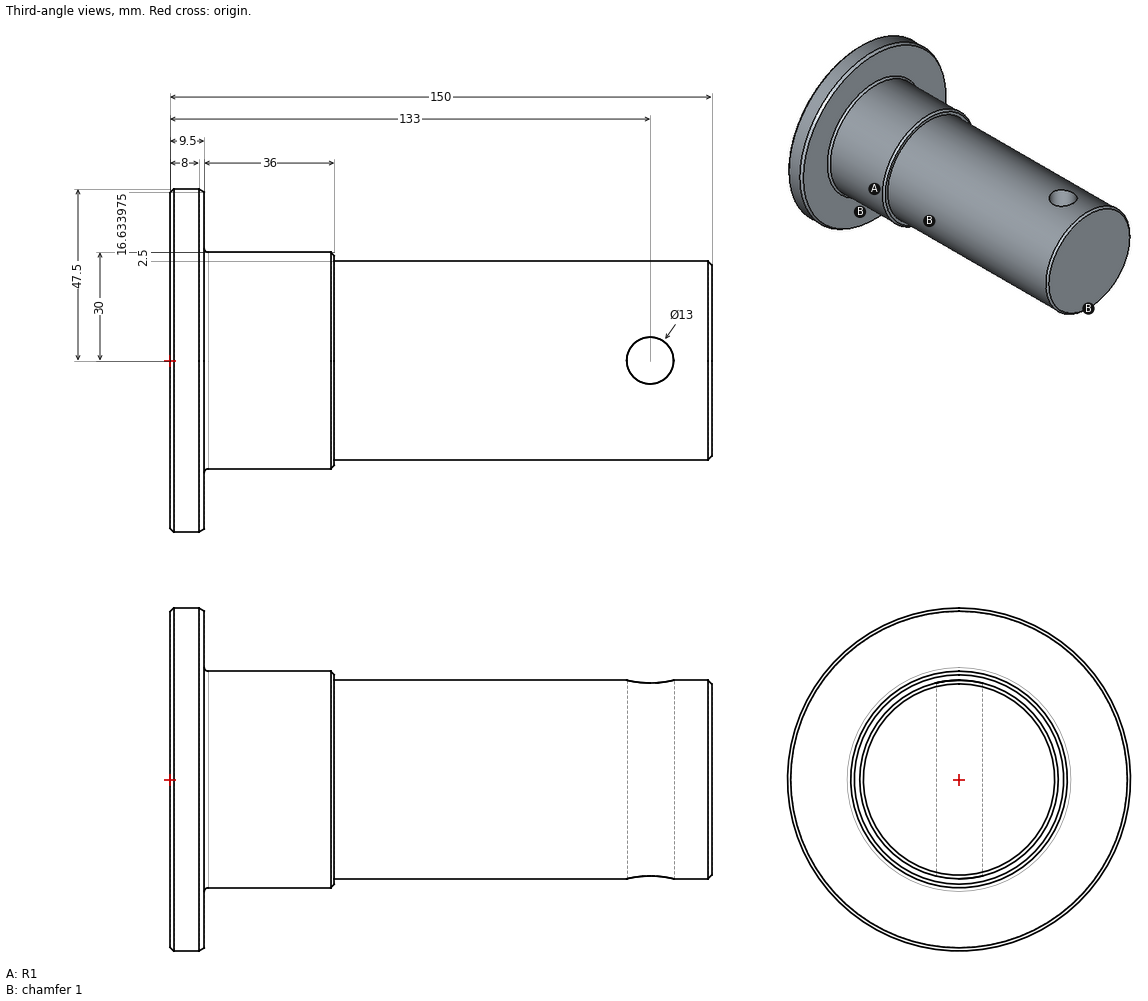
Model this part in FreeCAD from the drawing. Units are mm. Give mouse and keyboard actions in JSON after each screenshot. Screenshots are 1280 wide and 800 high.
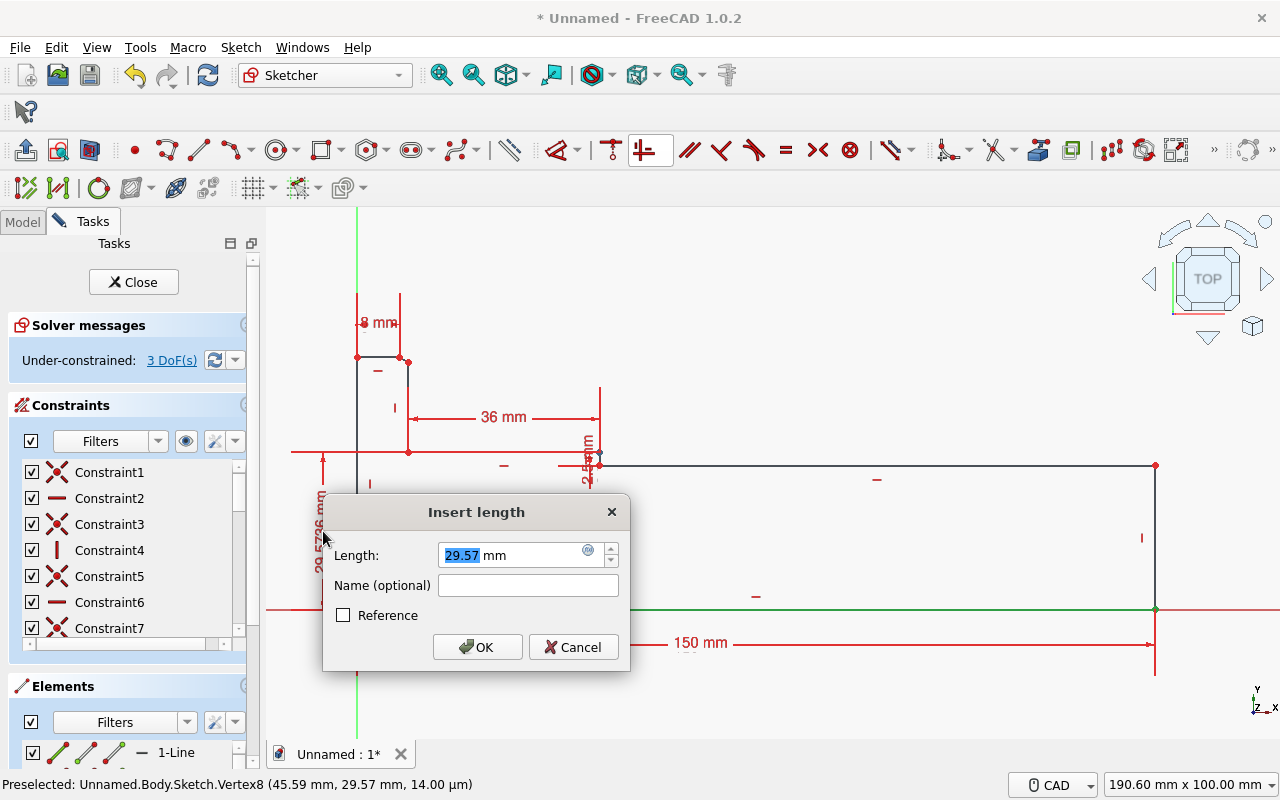
{"action": "type", "text": "30"}
{"action": "key", "text": "Return"}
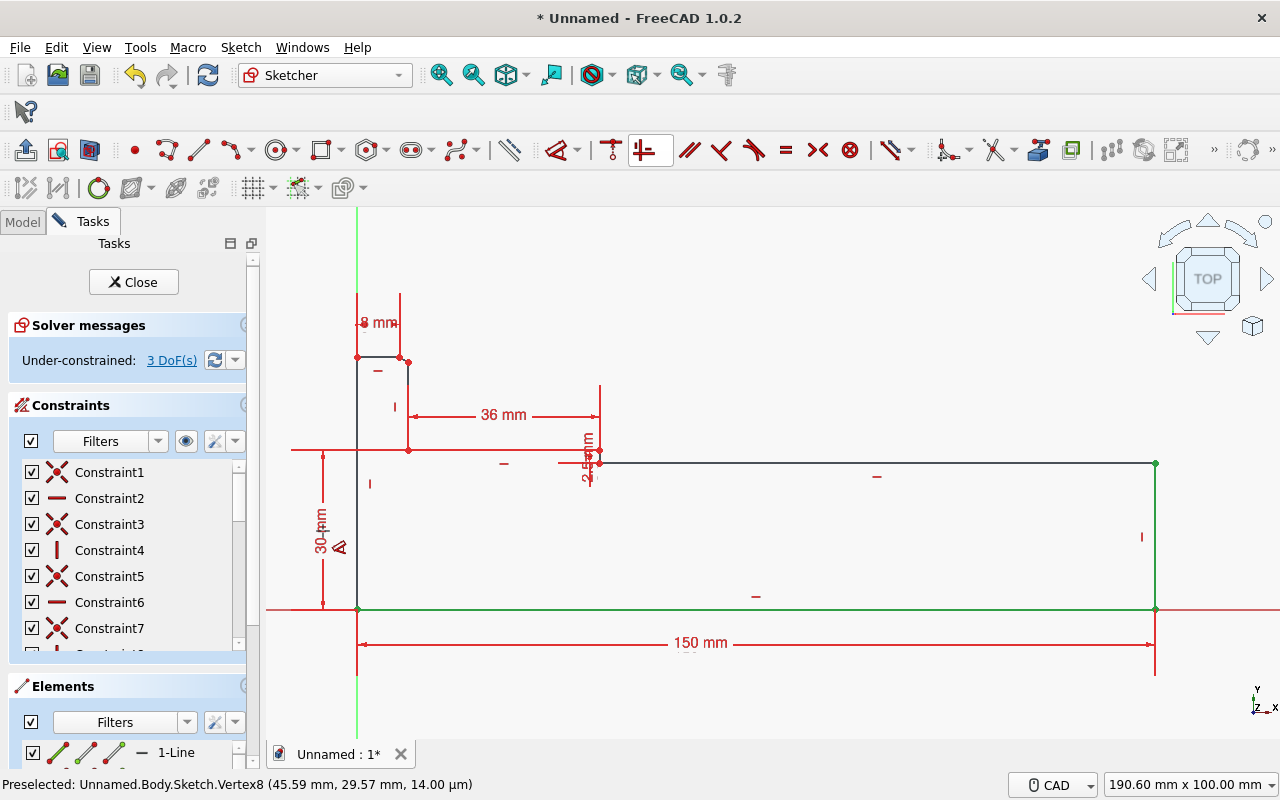
{"action": "left_click", "coordinate": [357, 433]}
{"action": "left_click", "coordinate": [323, 484]}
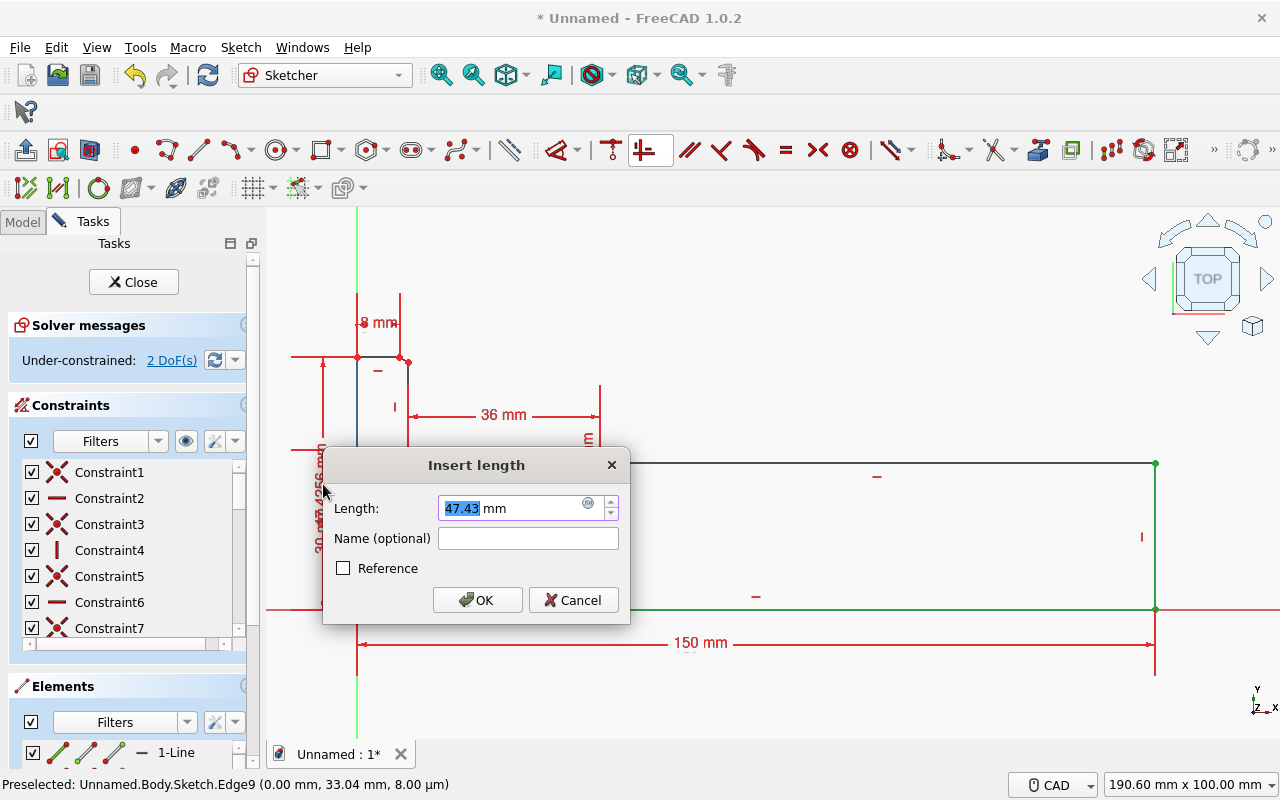
{"action": "type", "text": "47.5"}
{"action": "key", "text": "Return"}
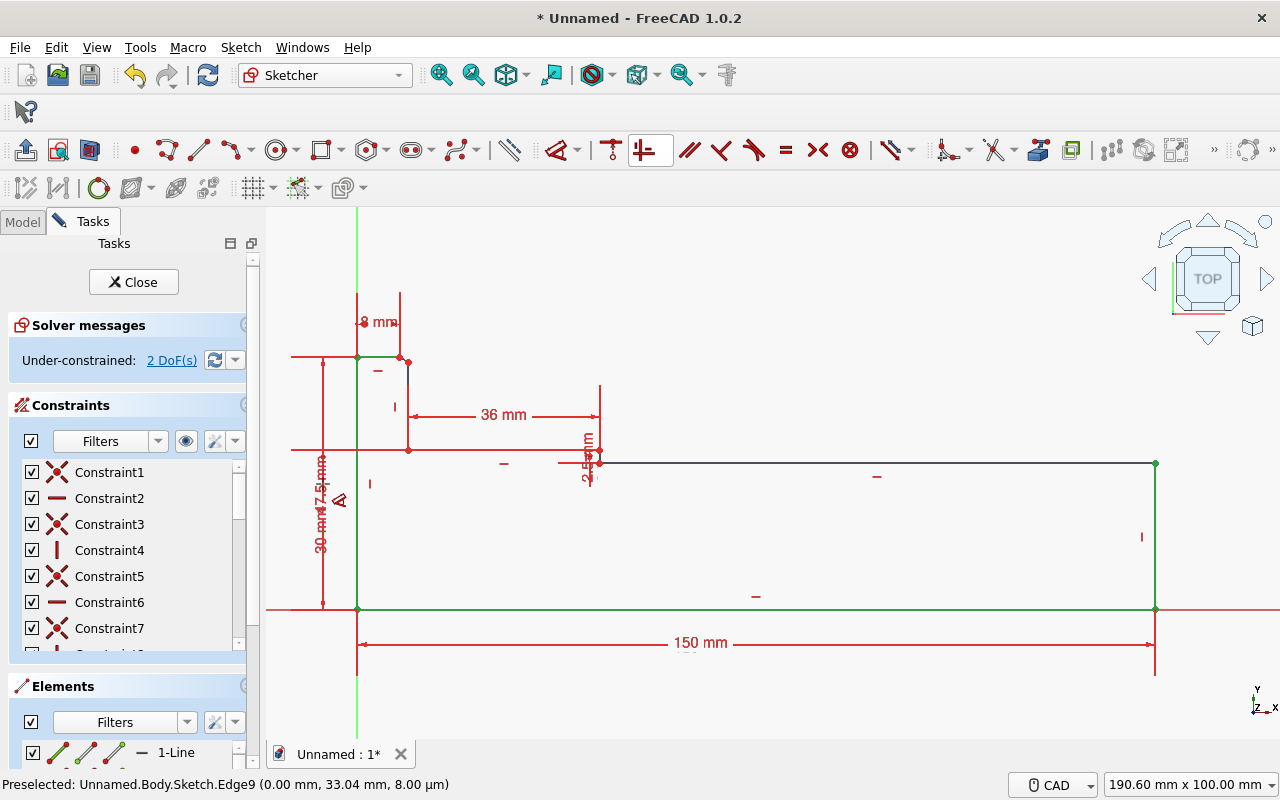
{"action": "left_click", "coordinate": [408, 450]}
{"action": "left_click", "coordinate": [383, 644]}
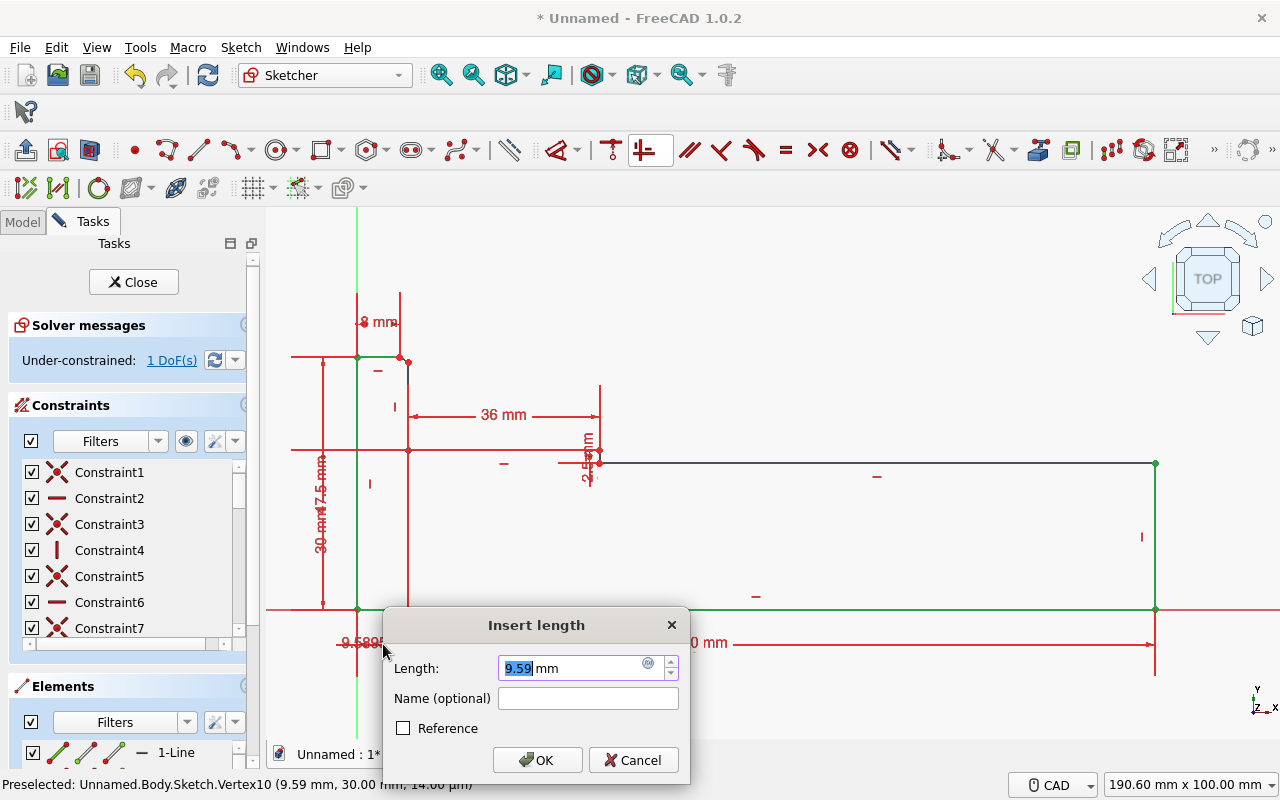
{"action": "type", "text": "9.5"}
{"action": "key", "text": "Return"}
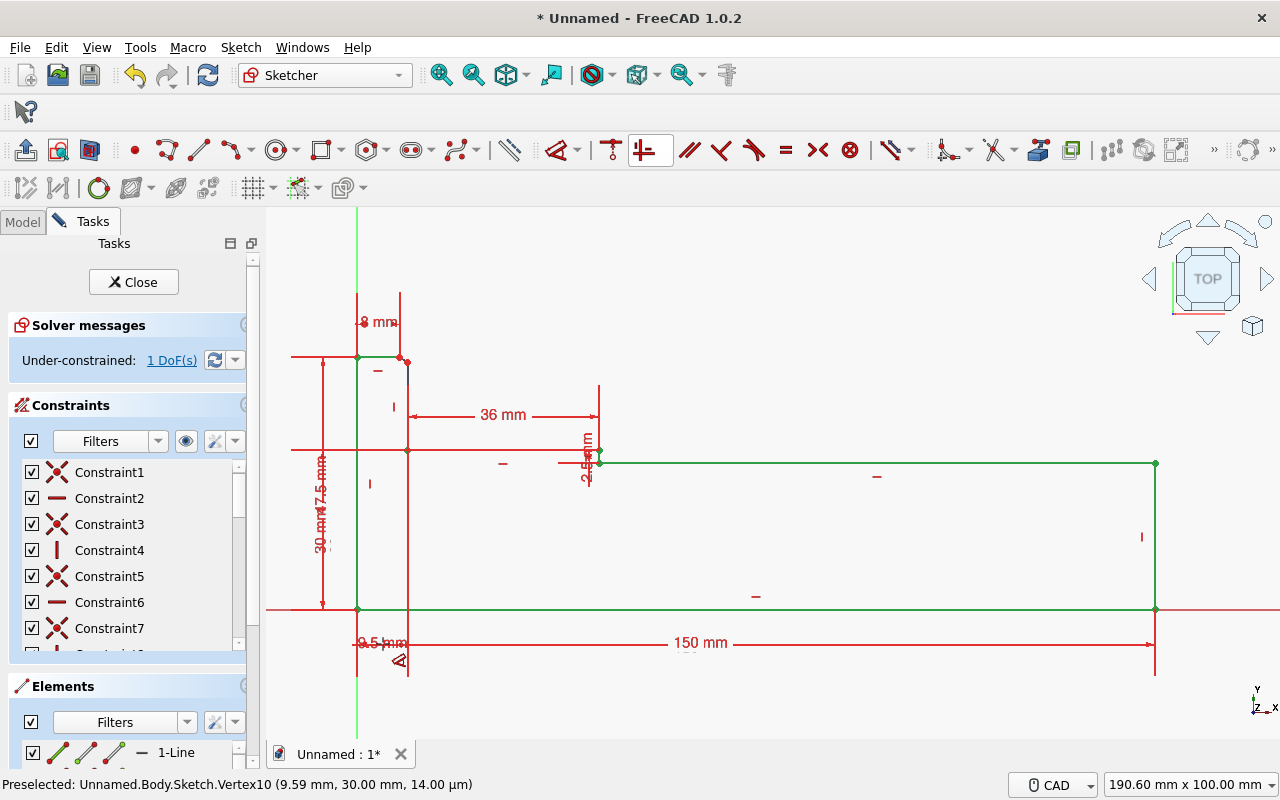
{"action": "left_click", "coordinate": [408, 424]}
{"action": "left_click", "coordinate": [374, 406]}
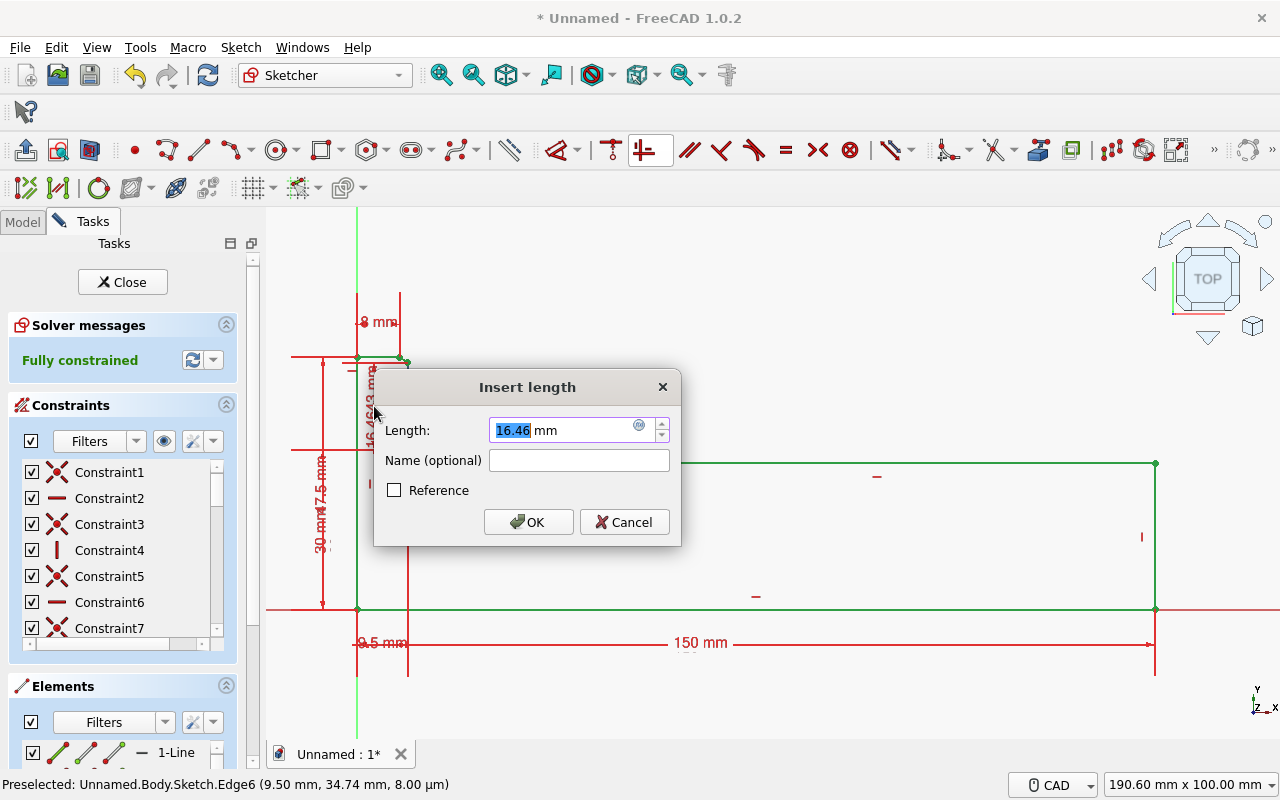
{"action": "type", "text": "16.633975"}
{"action": "key", "text": "Return"}
{"action": "key", "text": "Escape"}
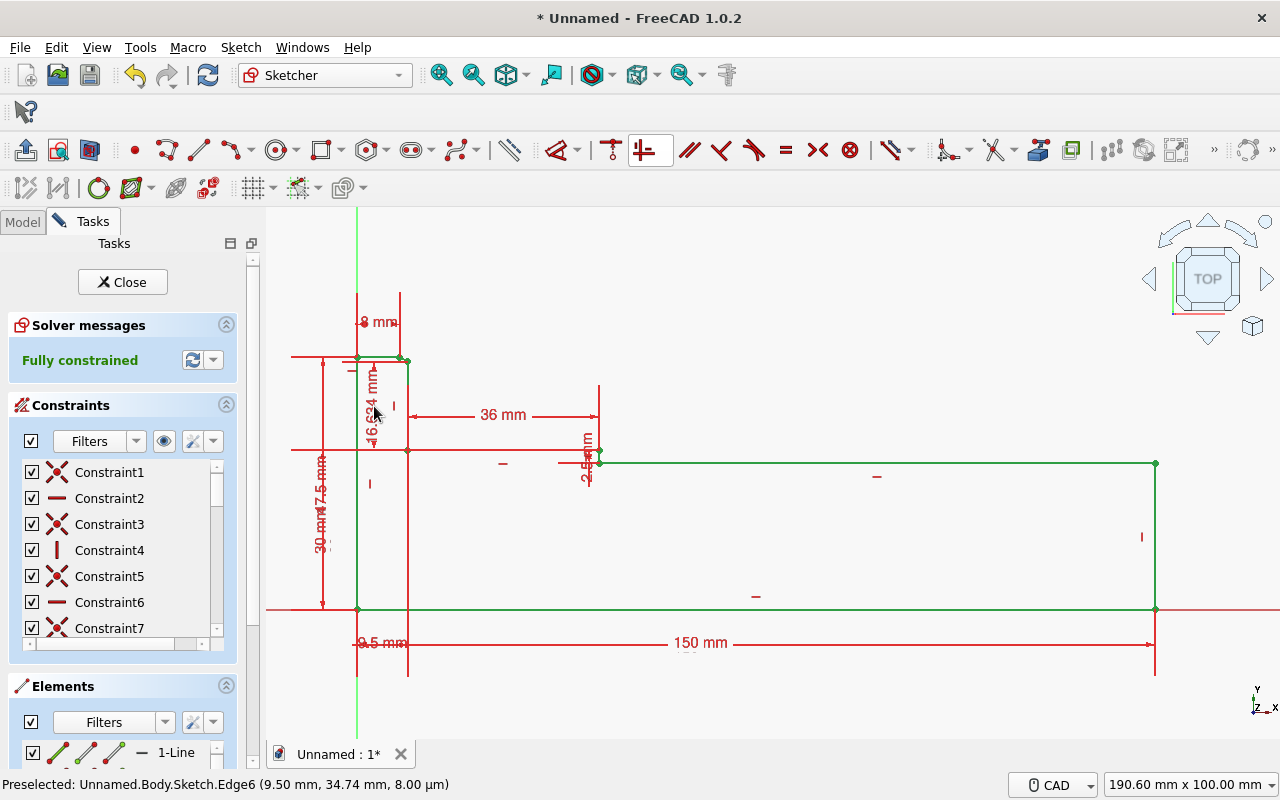
{"action": "left_click", "coordinate": [123, 282]}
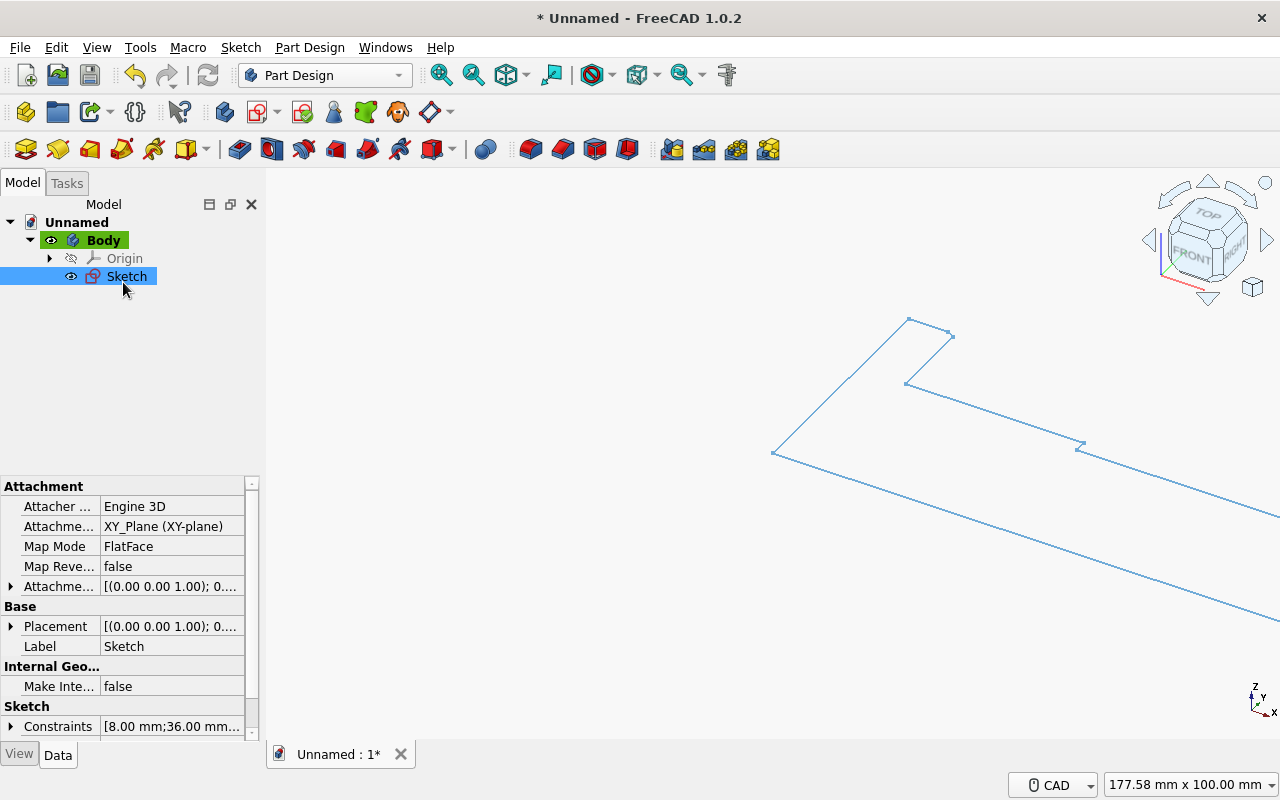
{"action": "left_click", "coordinate": [58, 150]}